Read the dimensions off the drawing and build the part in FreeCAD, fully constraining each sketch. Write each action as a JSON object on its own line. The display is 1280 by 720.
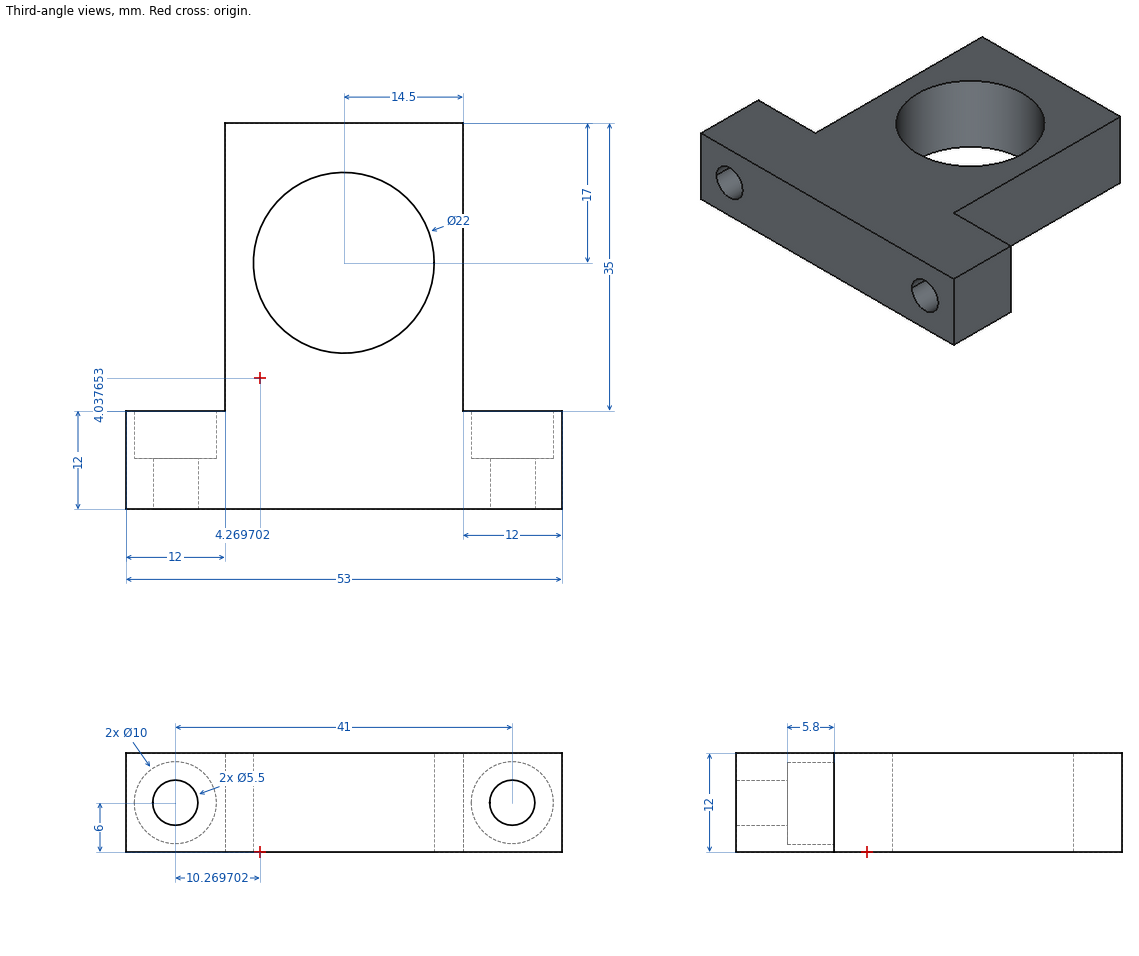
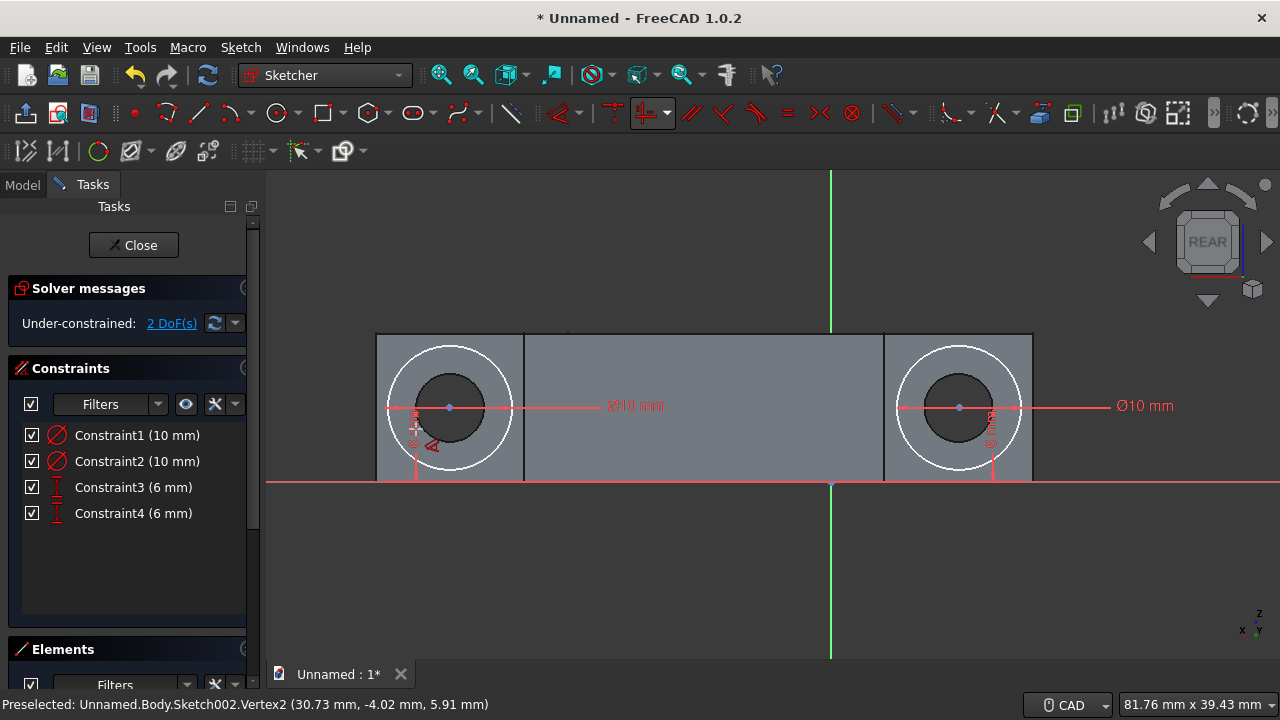
{"action": "left_click", "coordinate": [959, 408]}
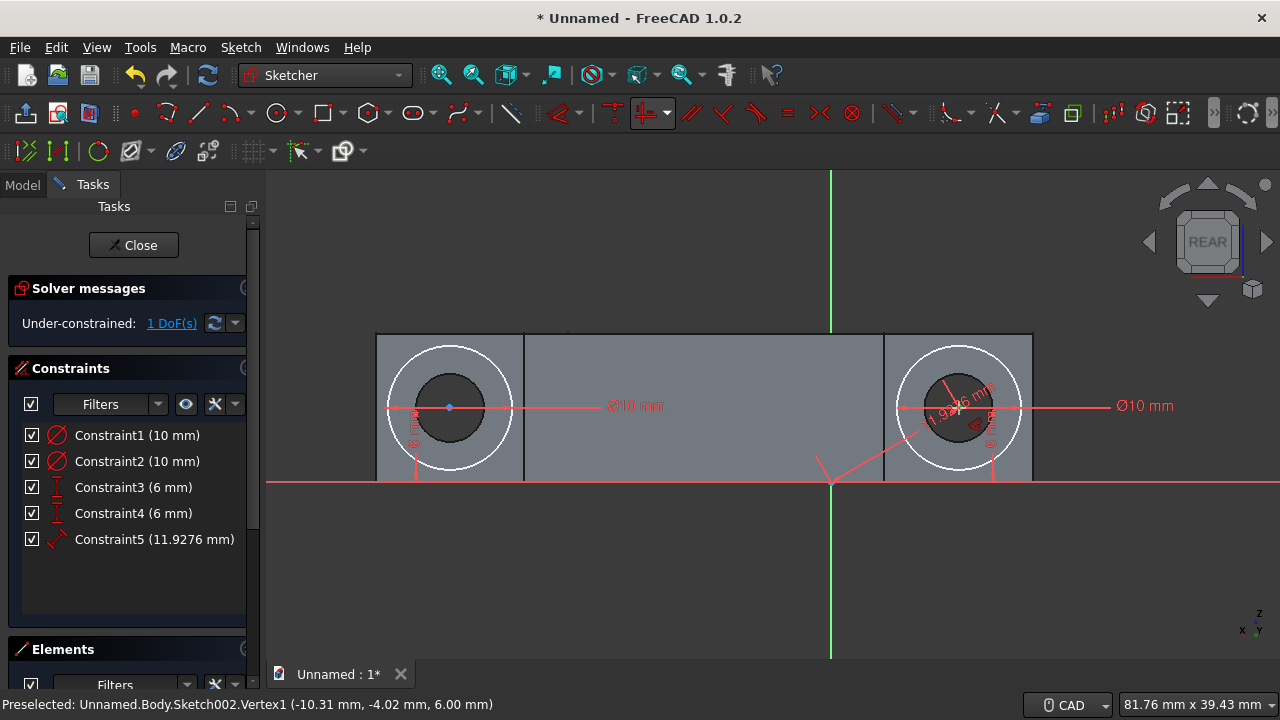
{"action": "left_click", "coordinate": [450, 408]}
{"action": "left_click", "coordinate": [704, 374]}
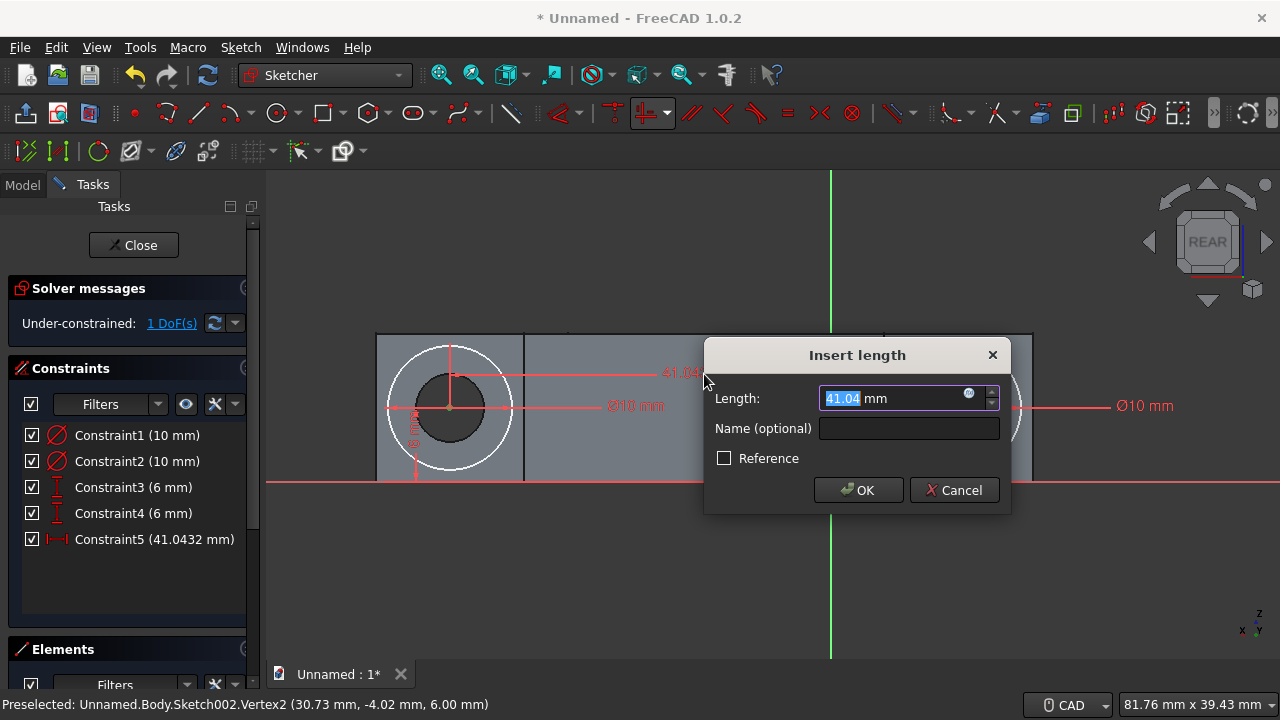
{"action": "type", "text": "41"}
{"action": "key", "text": "Return"}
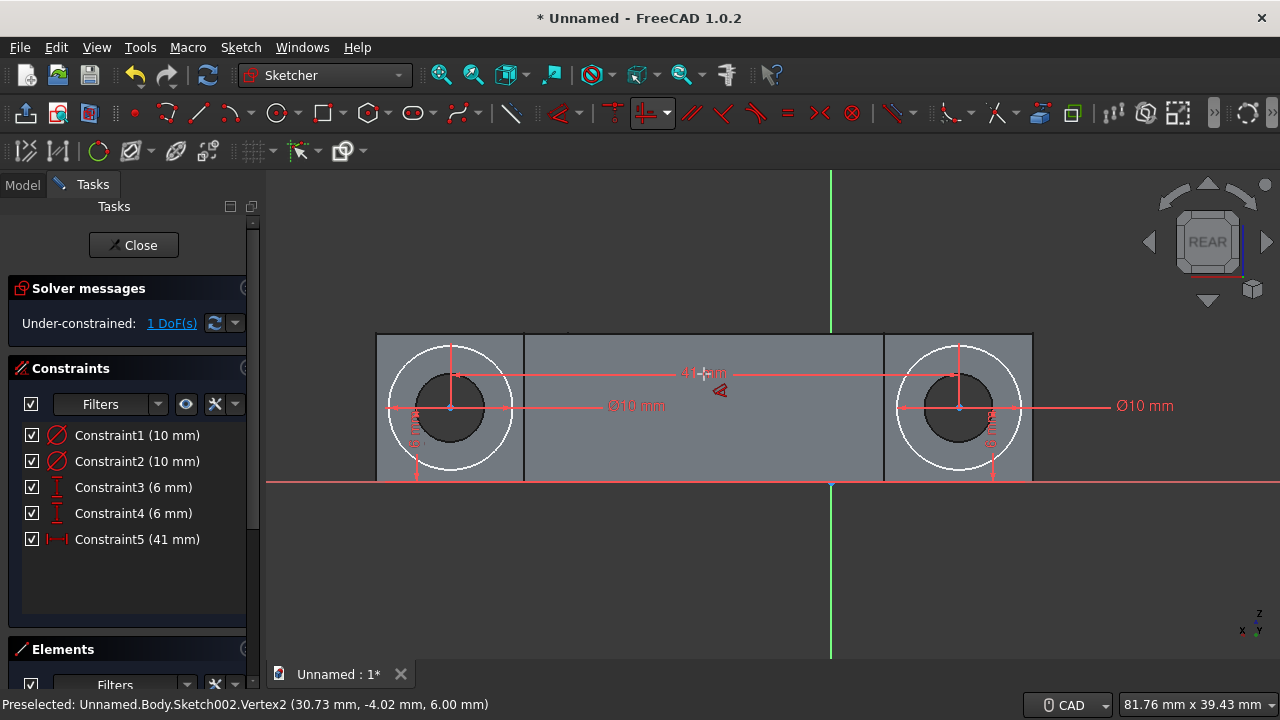
{"action": "left_click", "coordinate": [959, 408]}
{"action": "left_click", "coordinate": [895, 516]}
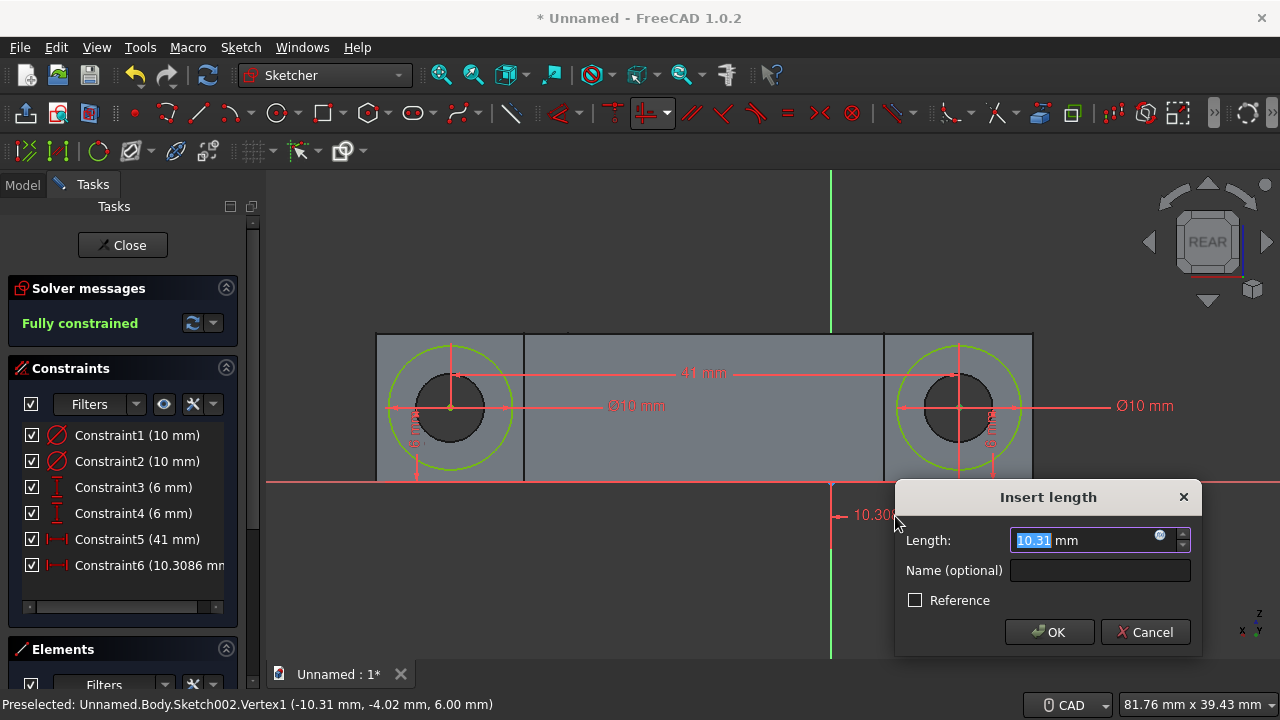
{"action": "type", "text": "10.269702"}
{"action": "key", "text": "Return"}
{"action": "key", "text": "Escape"}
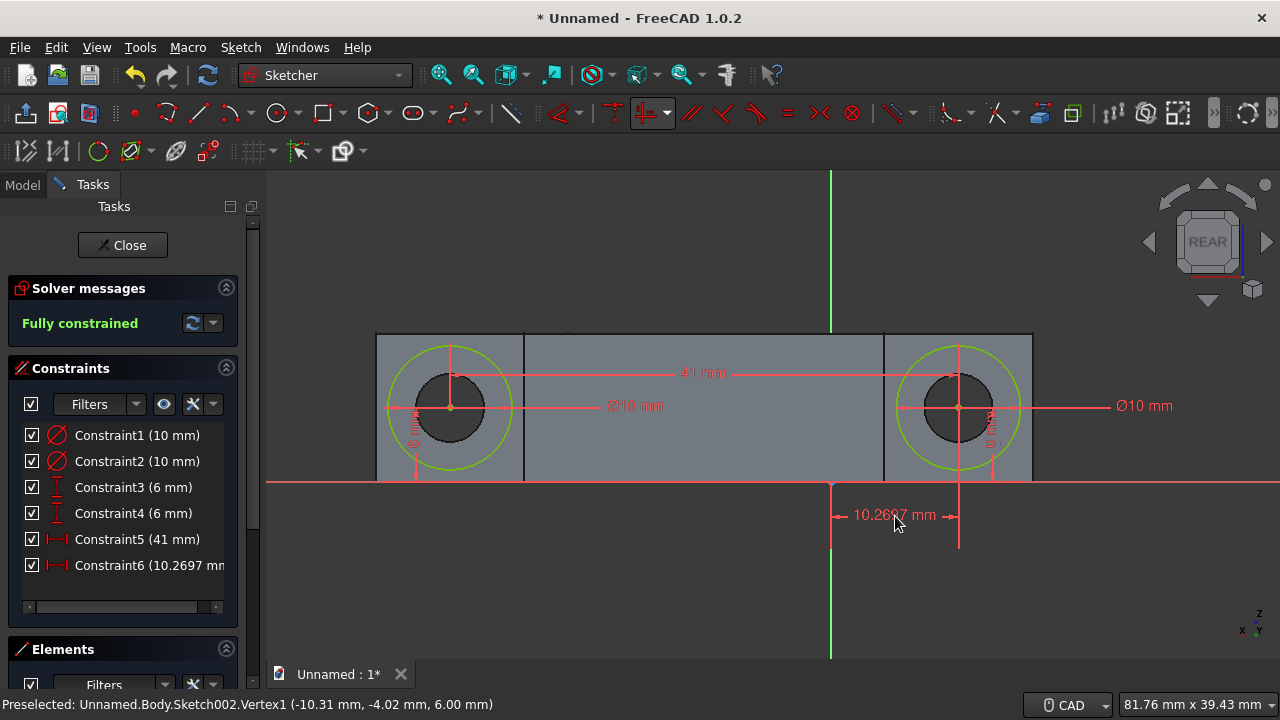
{"action": "left_click", "coordinate": [123, 245]}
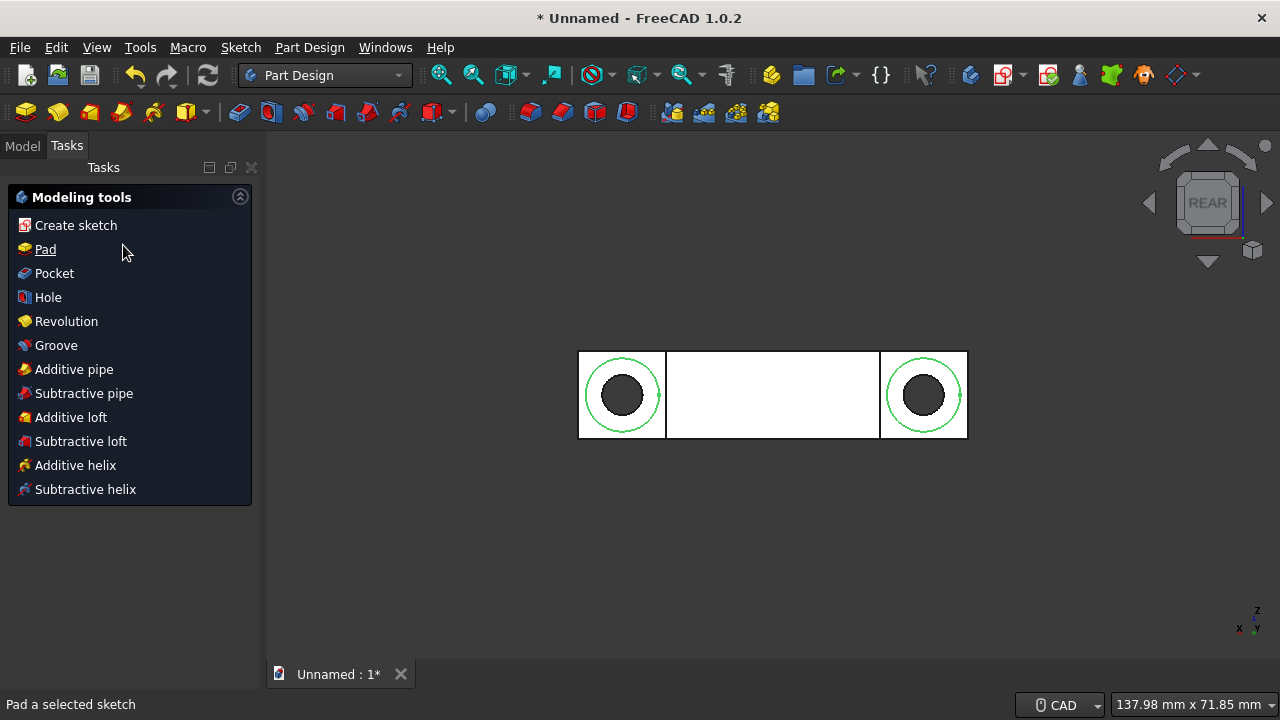
{"action": "left_click", "coordinate": [240, 112]}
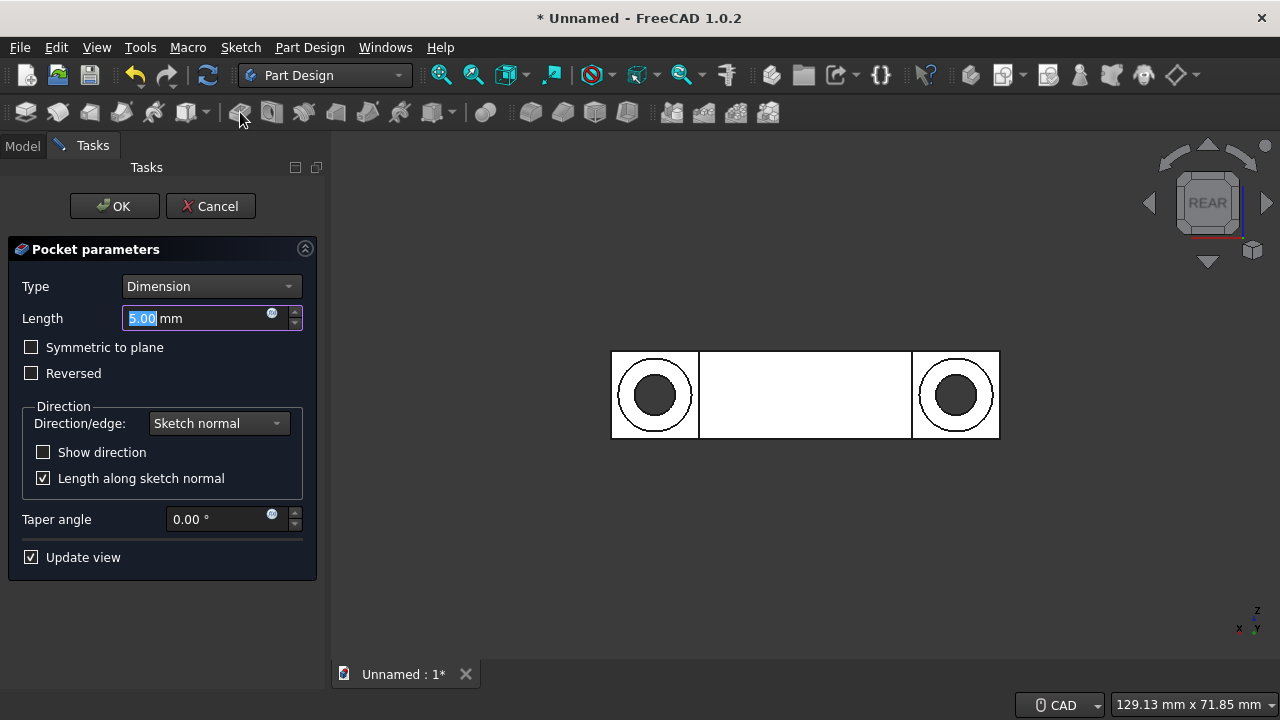
{"action": "type", "text": "5.8"}
{"action": "key", "text": "Tab"}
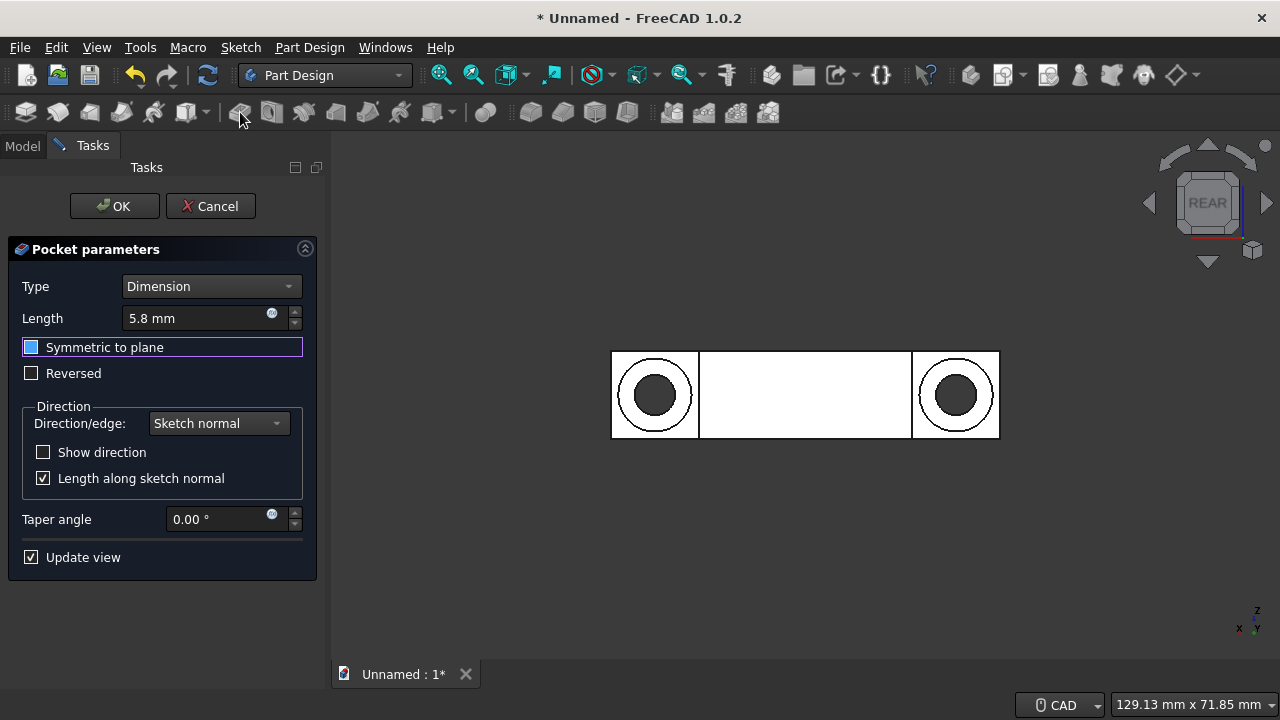
{"action": "left_click", "coordinate": [115, 206]}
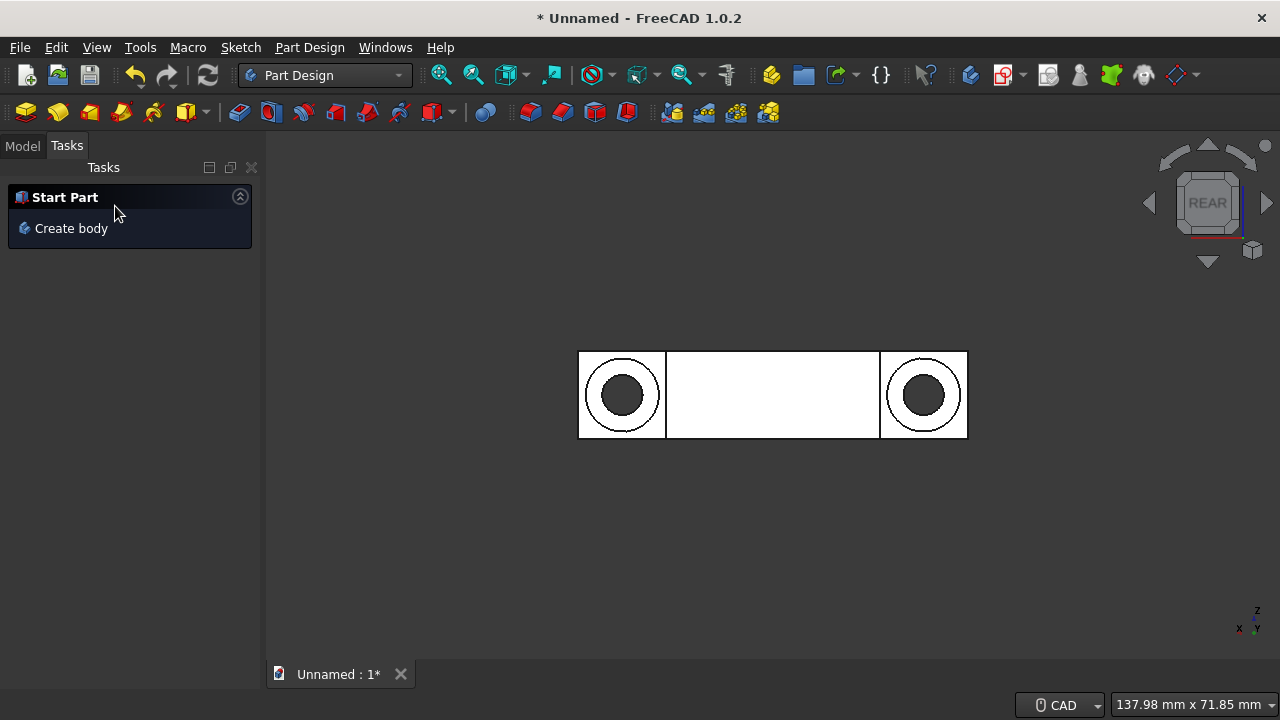
{"action": "key", "text": "0"}